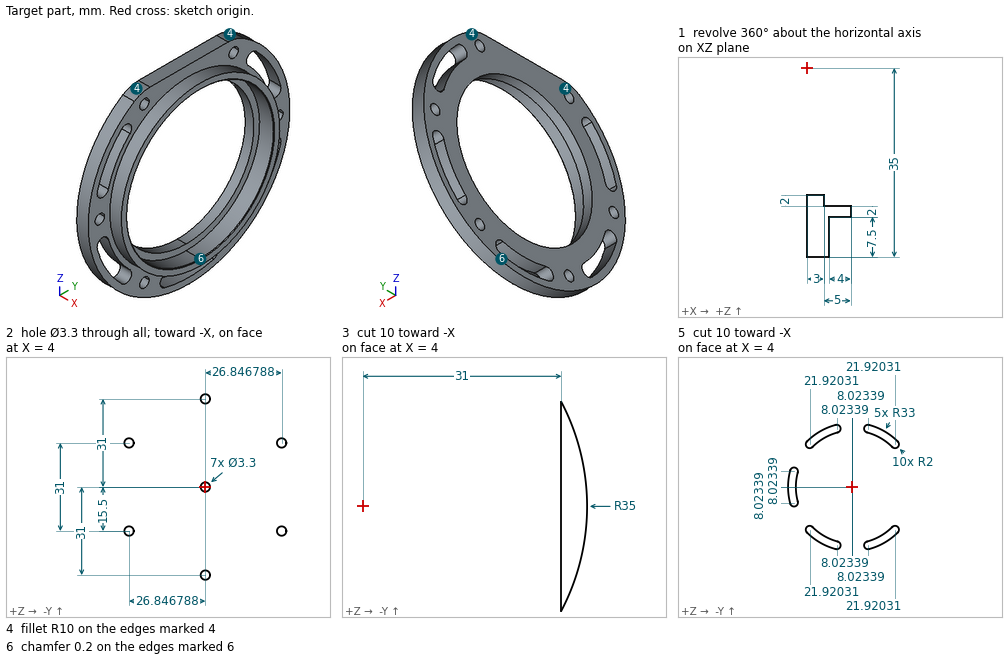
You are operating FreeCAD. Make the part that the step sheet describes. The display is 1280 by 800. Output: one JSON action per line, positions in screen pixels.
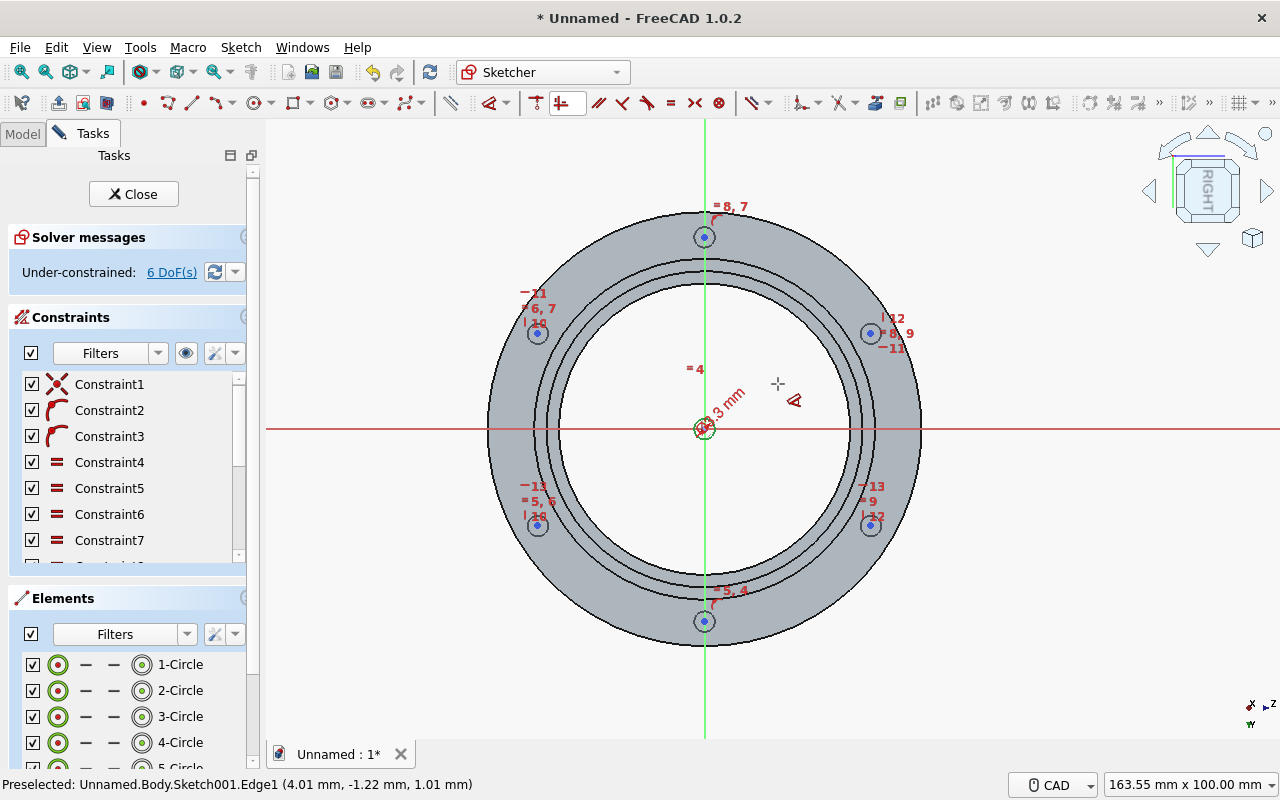
{"action": "left_click", "coordinate": [705, 622]}
{"action": "left_click", "coordinate": [739, 525]}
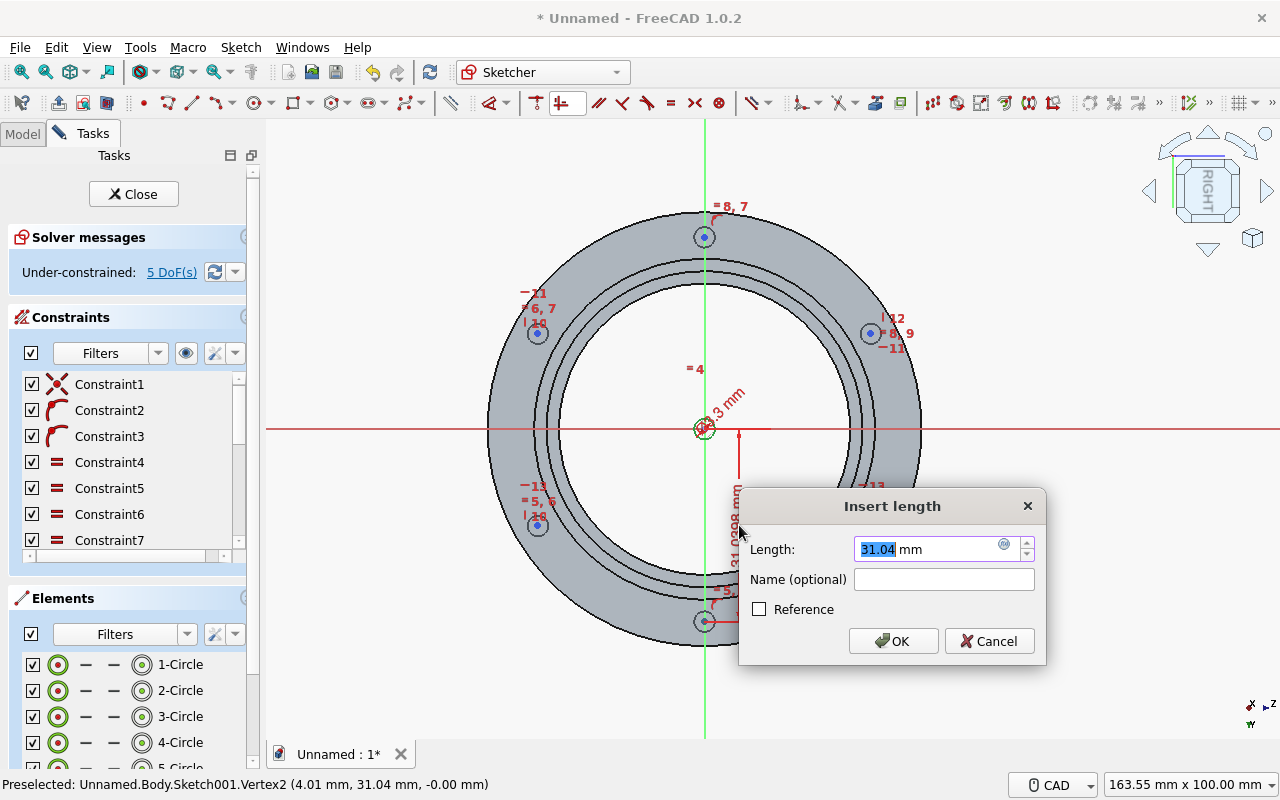
{"action": "type", "text": "31"}
{"action": "key", "text": "Return"}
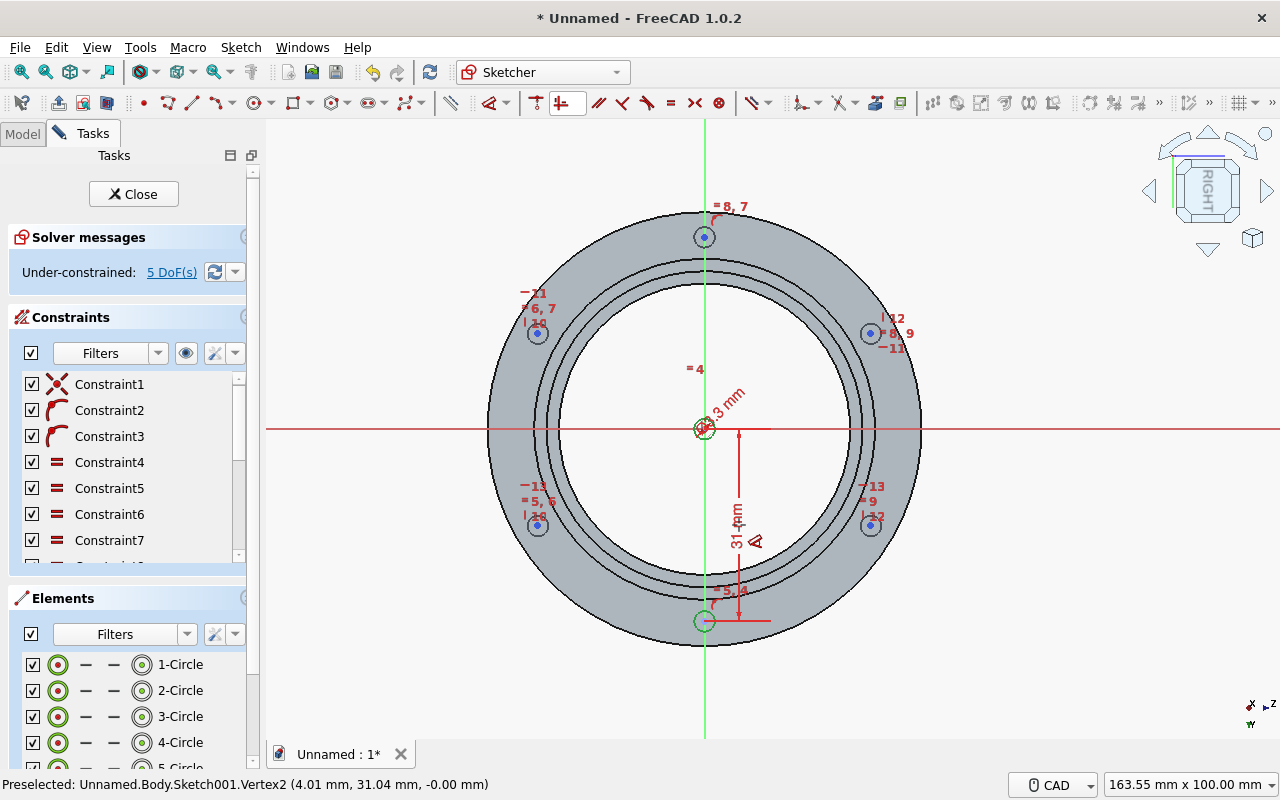
{"action": "left_click", "coordinate": [705, 237]}
{"action": "left_click", "coordinate": [739, 333]}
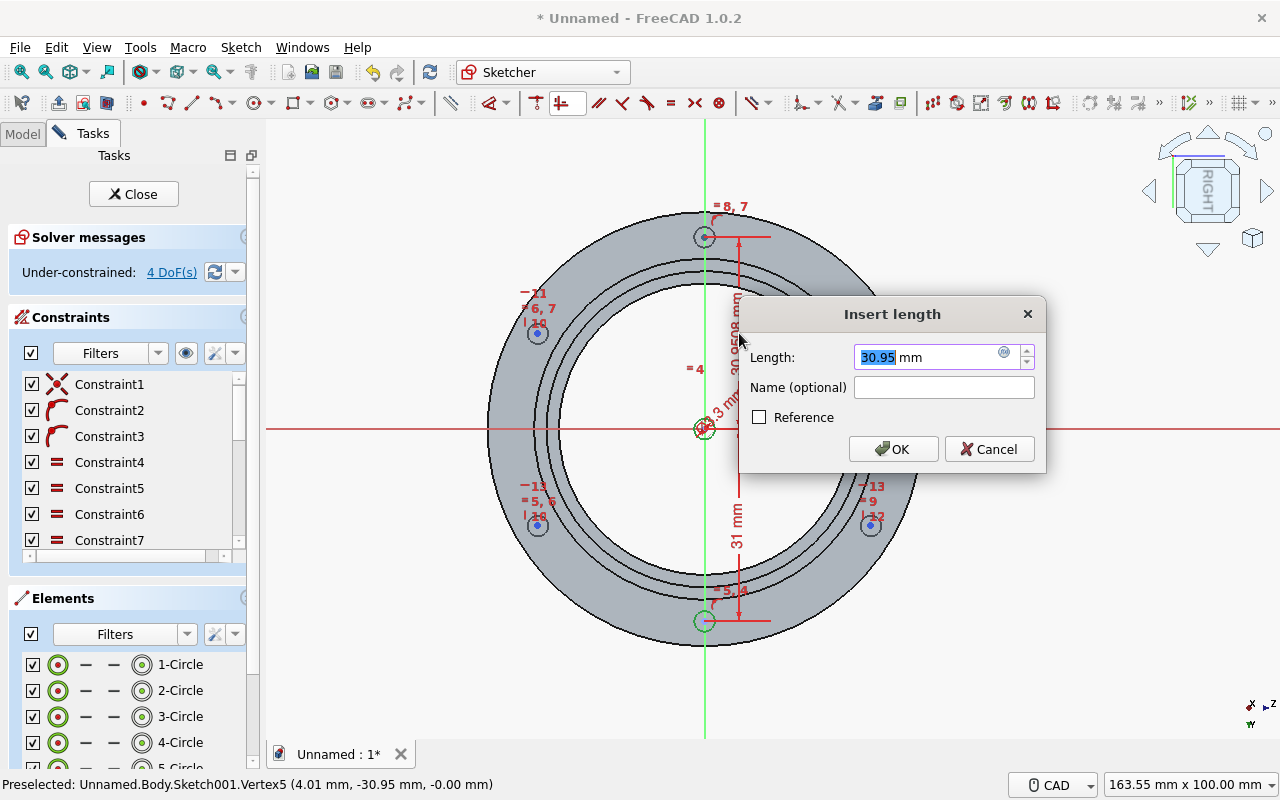
{"action": "type", "text": "31"}
{"action": "key", "text": "Return"}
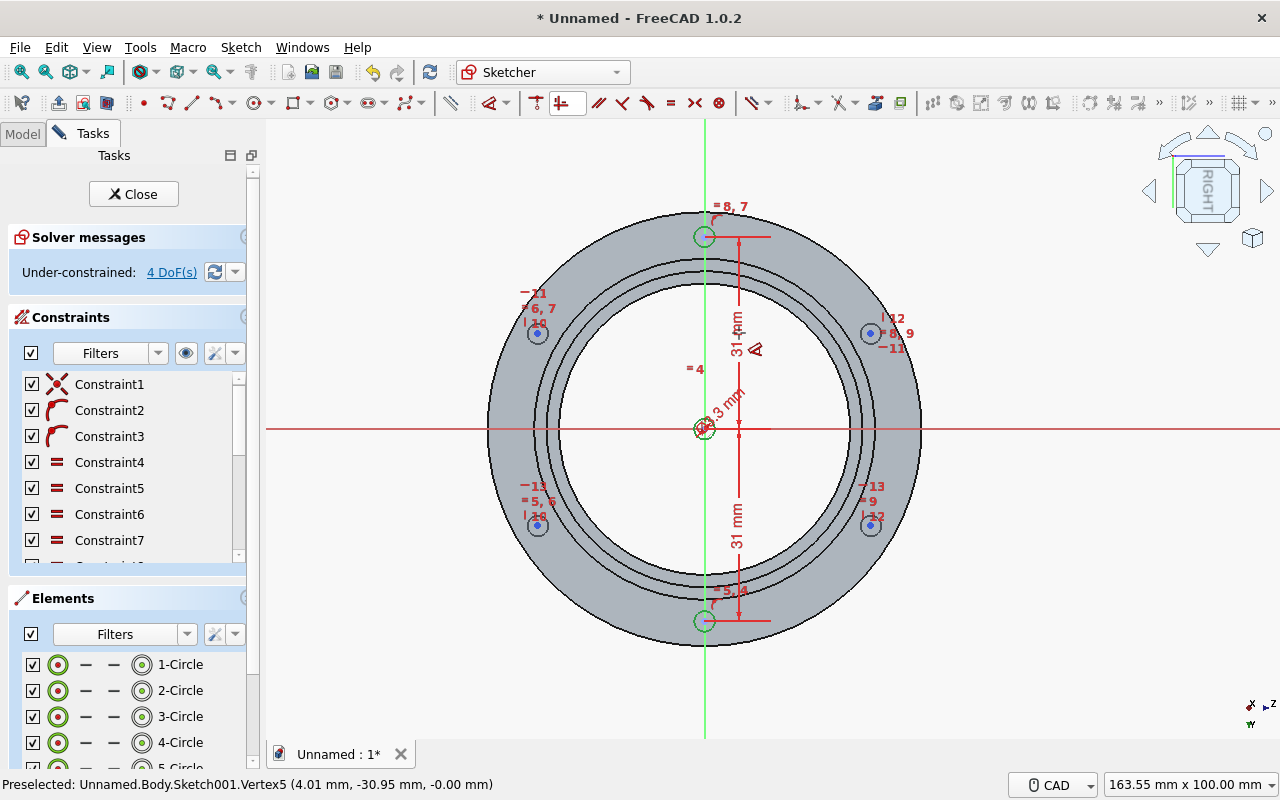
{"action": "left_click", "coordinate": [538, 526]}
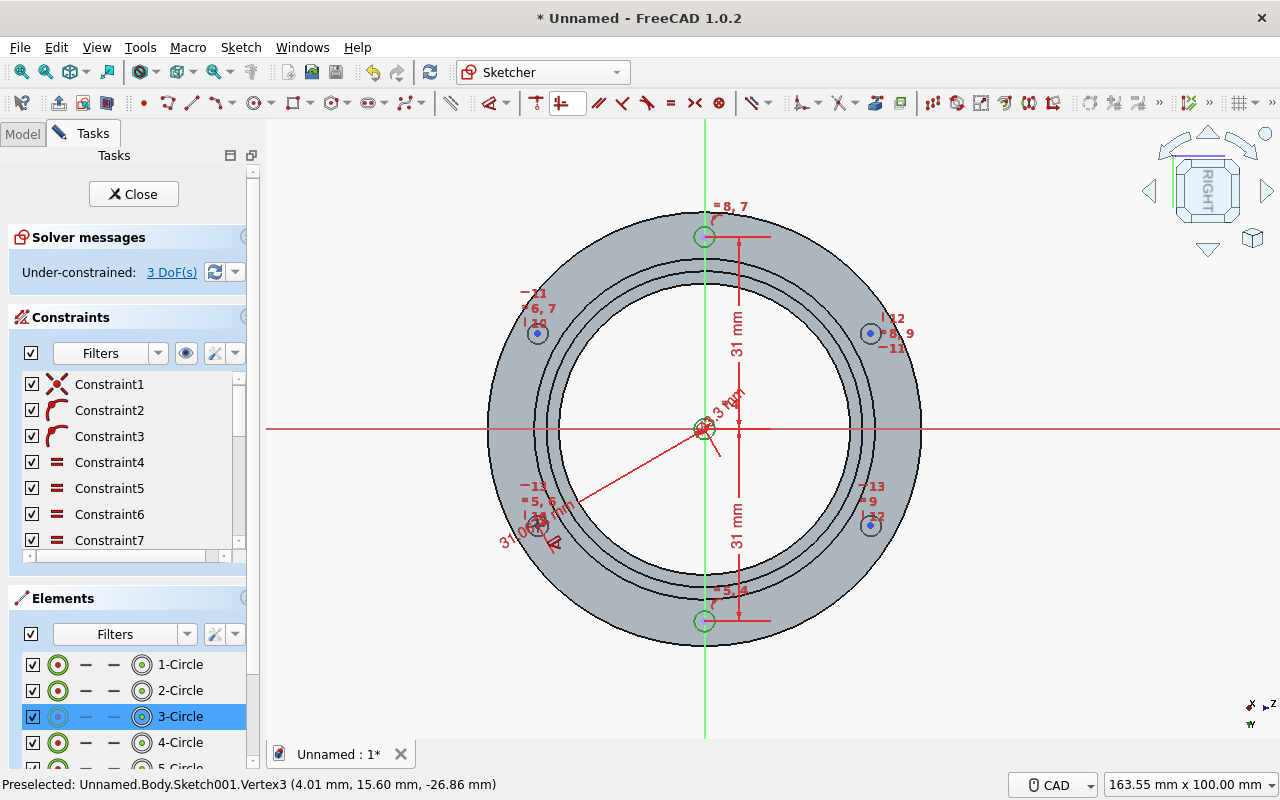
{"action": "left_click", "coordinate": [538, 334]}
{"action": "left_click", "coordinate": [504, 386]}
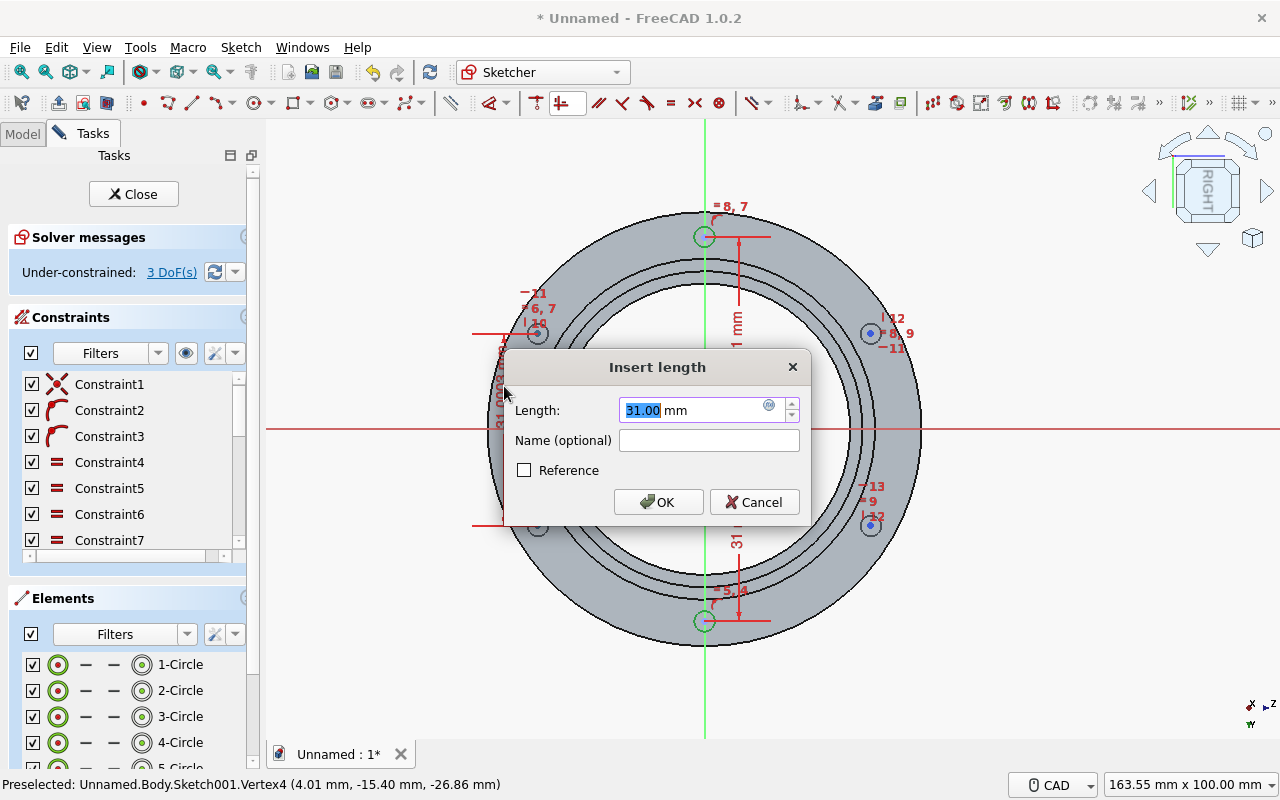
{"action": "type", "text": "31"}
{"action": "key", "text": "Return"}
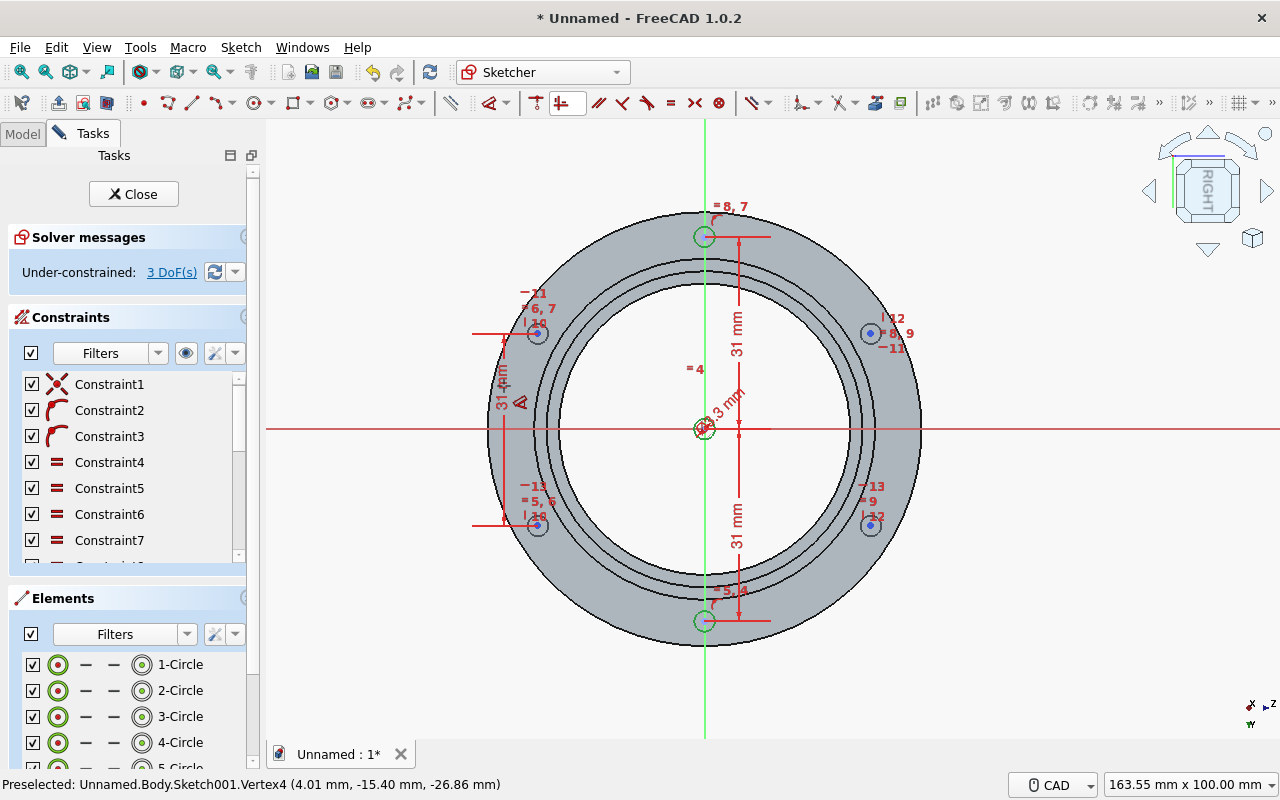
{"action": "left_click", "coordinate": [538, 526]}
{"action": "left_click", "coordinate": [504, 478]}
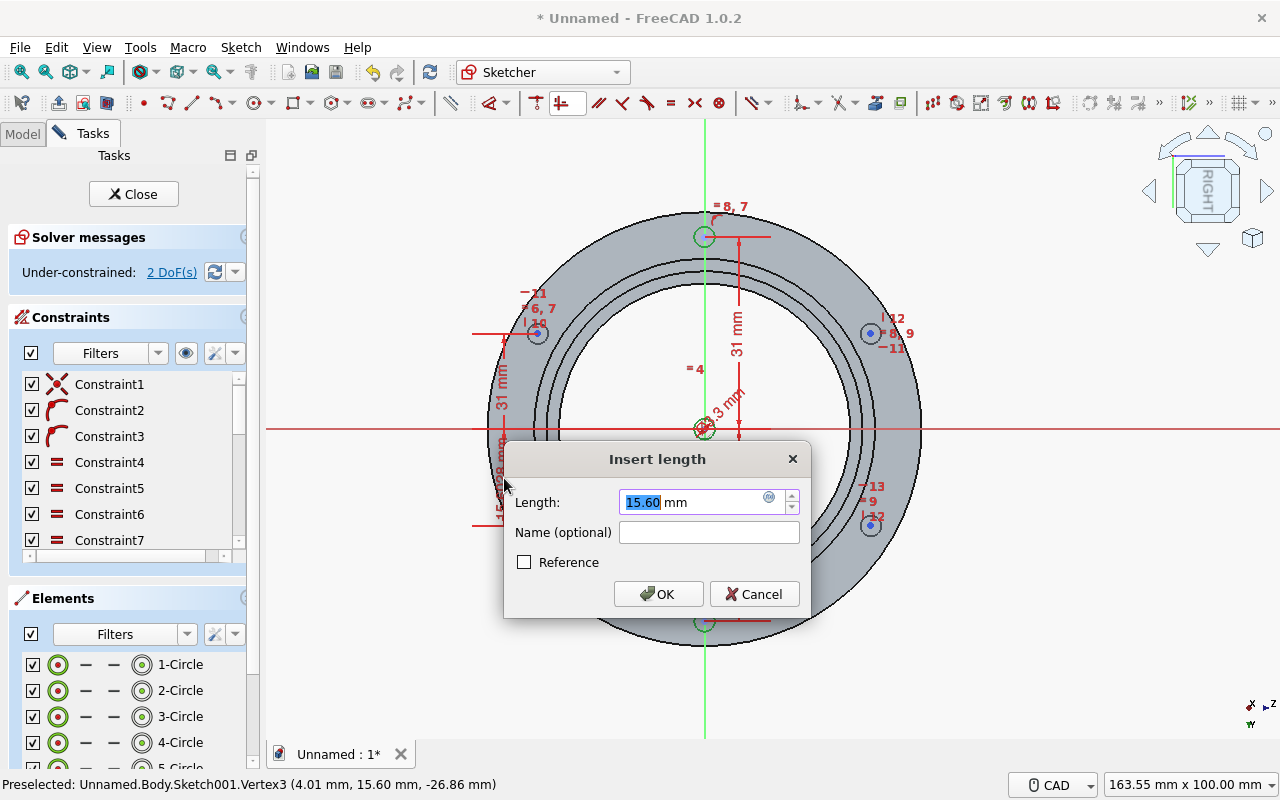
{"action": "type", "text": "15.5"}
{"action": "key", "text": "Return"}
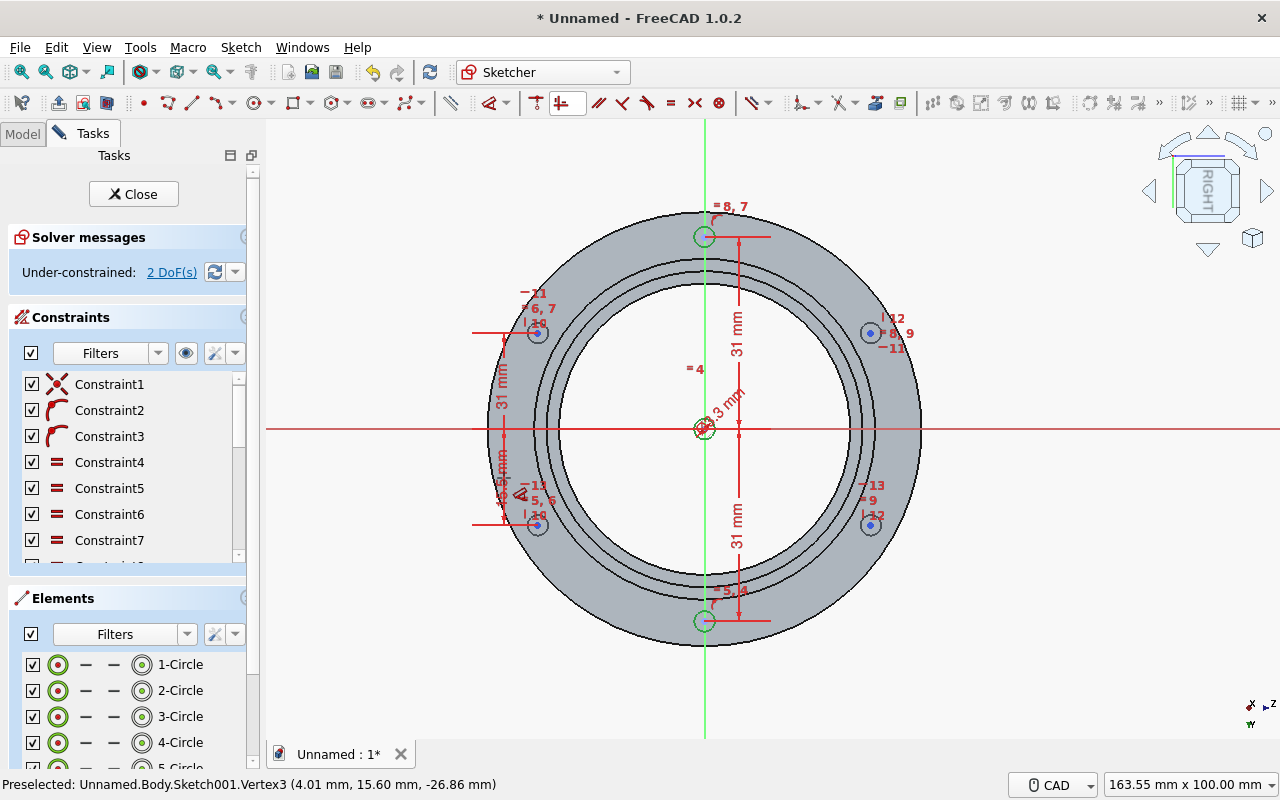
{"action": "left_click", "coordinate": [538, 525]}
{"action": "left_click", "coordinate": [621, 559]}